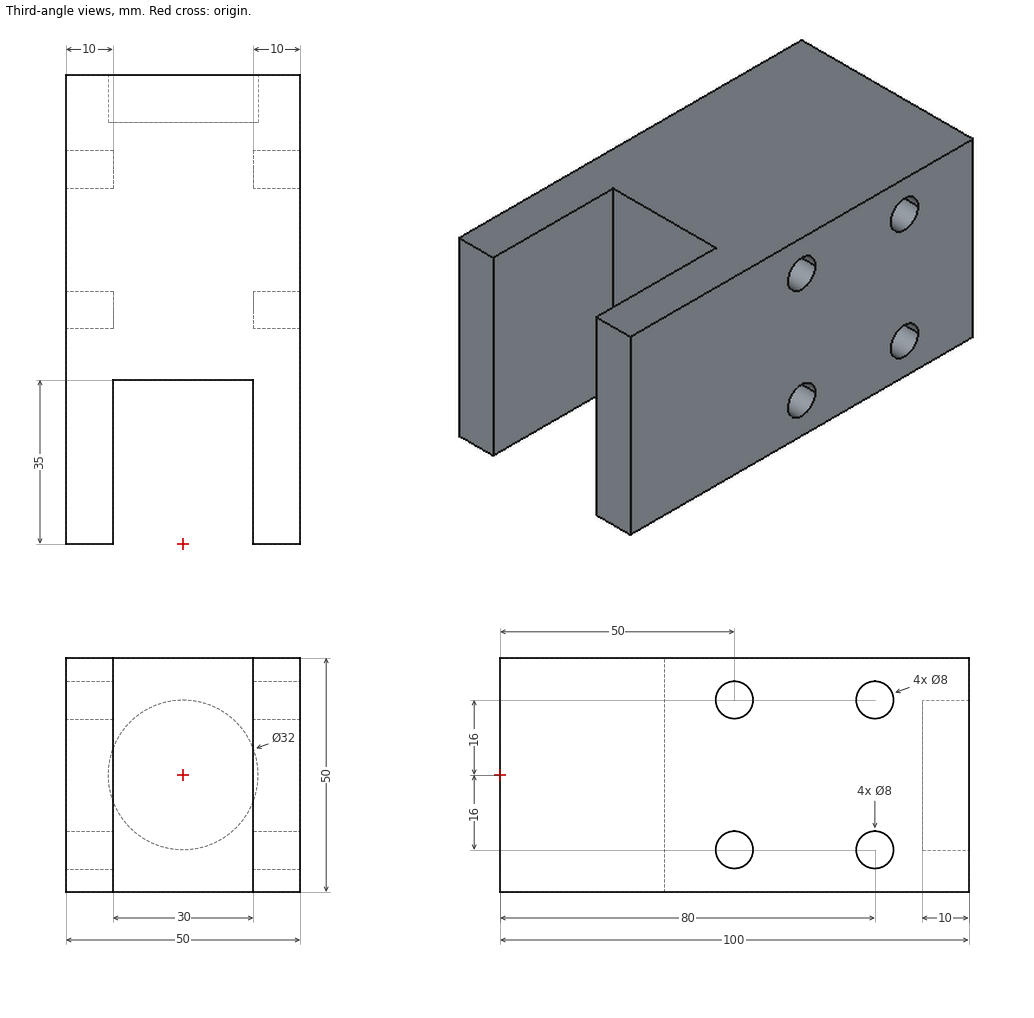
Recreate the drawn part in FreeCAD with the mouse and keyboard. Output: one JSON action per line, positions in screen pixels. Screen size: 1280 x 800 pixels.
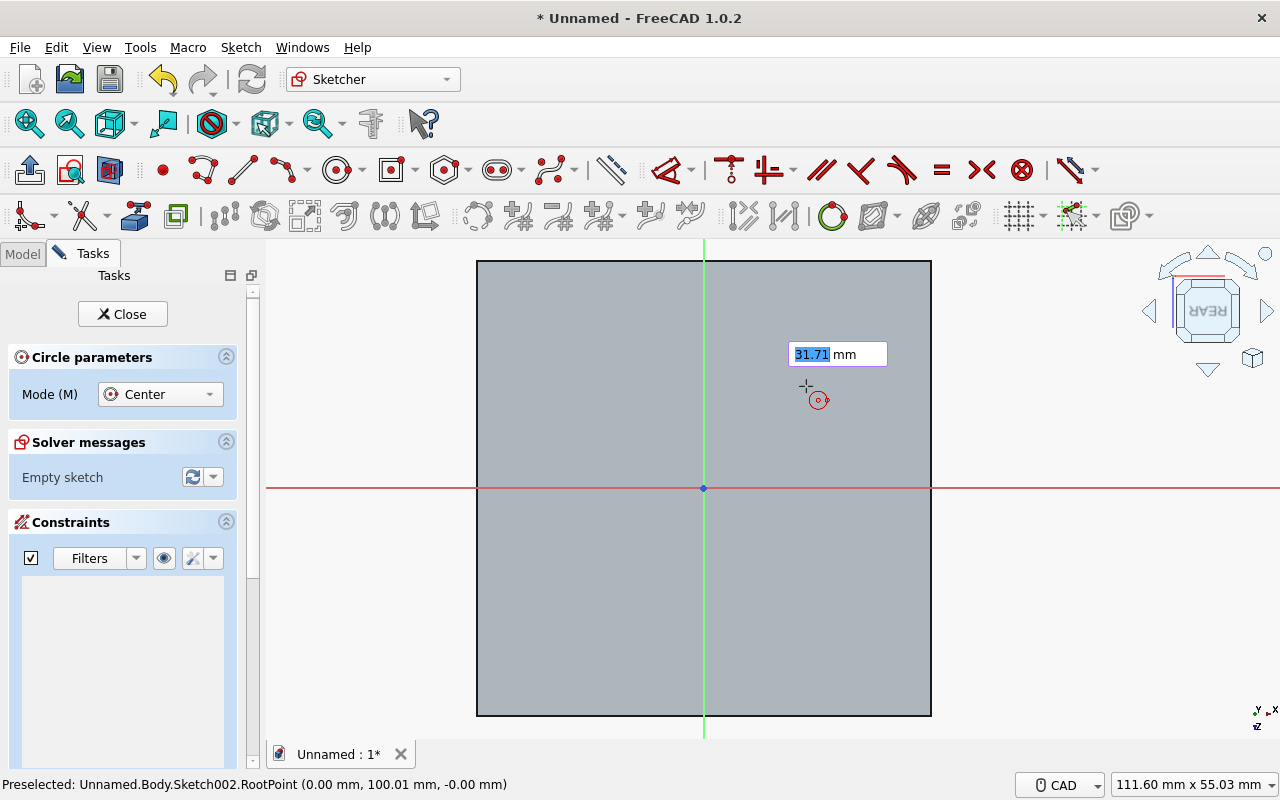
{"action": "type", "text": "32"}
{"action": "key", "text": "Return"}
{"action": "key", "text": "Escape"}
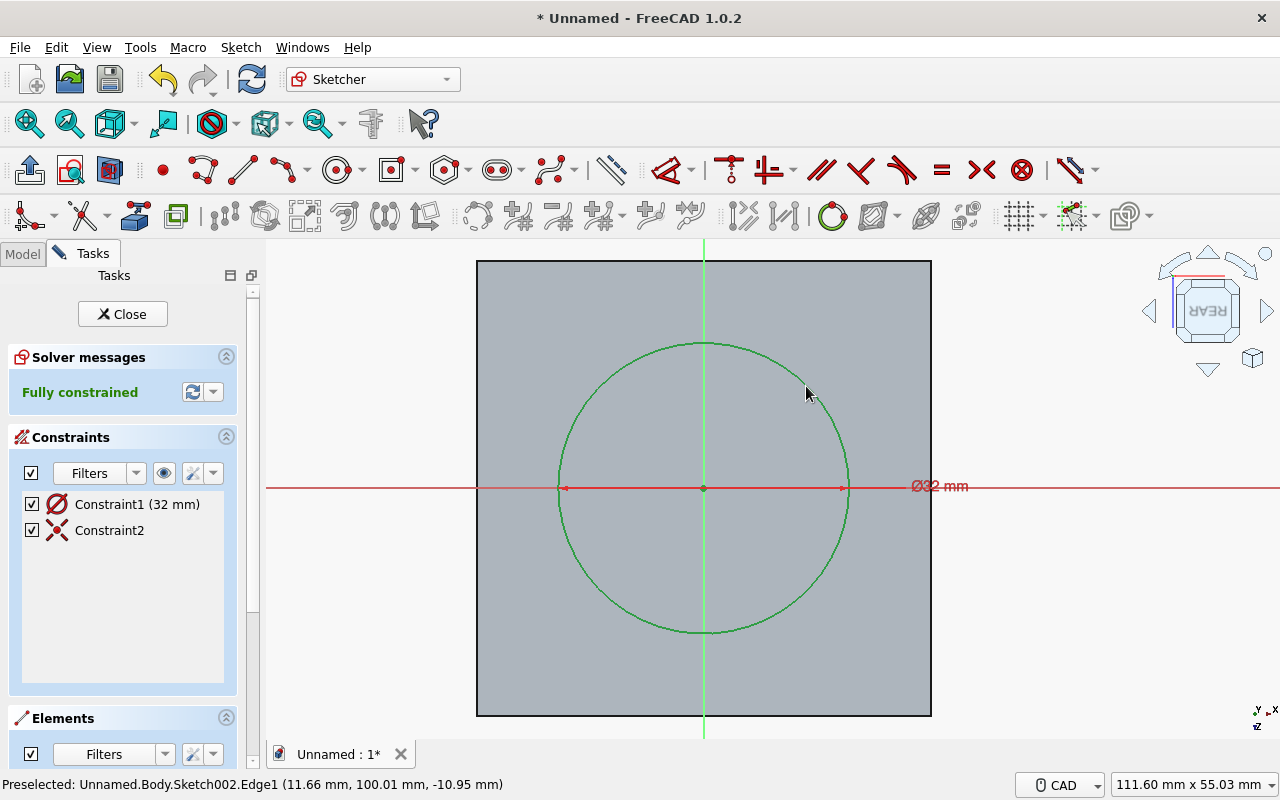
{"action": "left_click", "coordinate": [123, 314]}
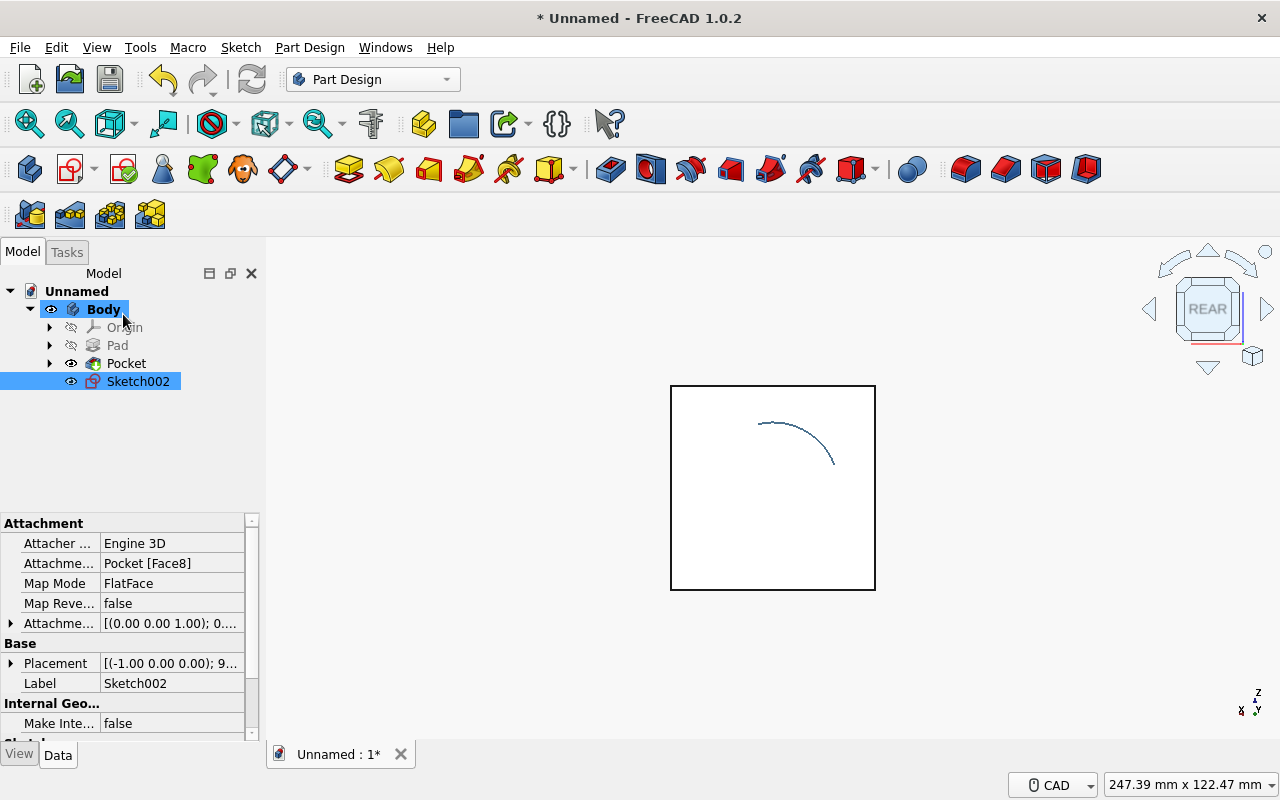
{"action": "left_click", "coordinate": [612, 170]}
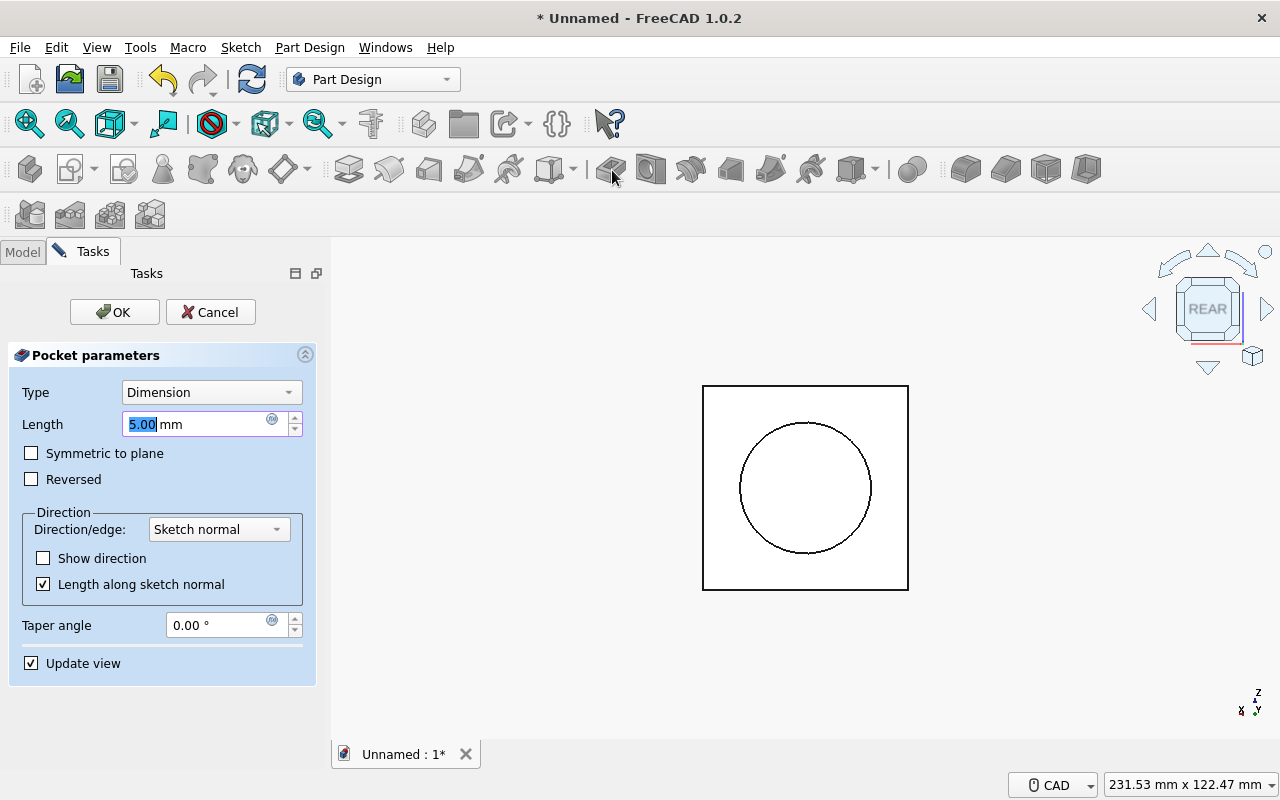
{"action": "type", "text": "10"}
{"action": "key", "text": "Tab"}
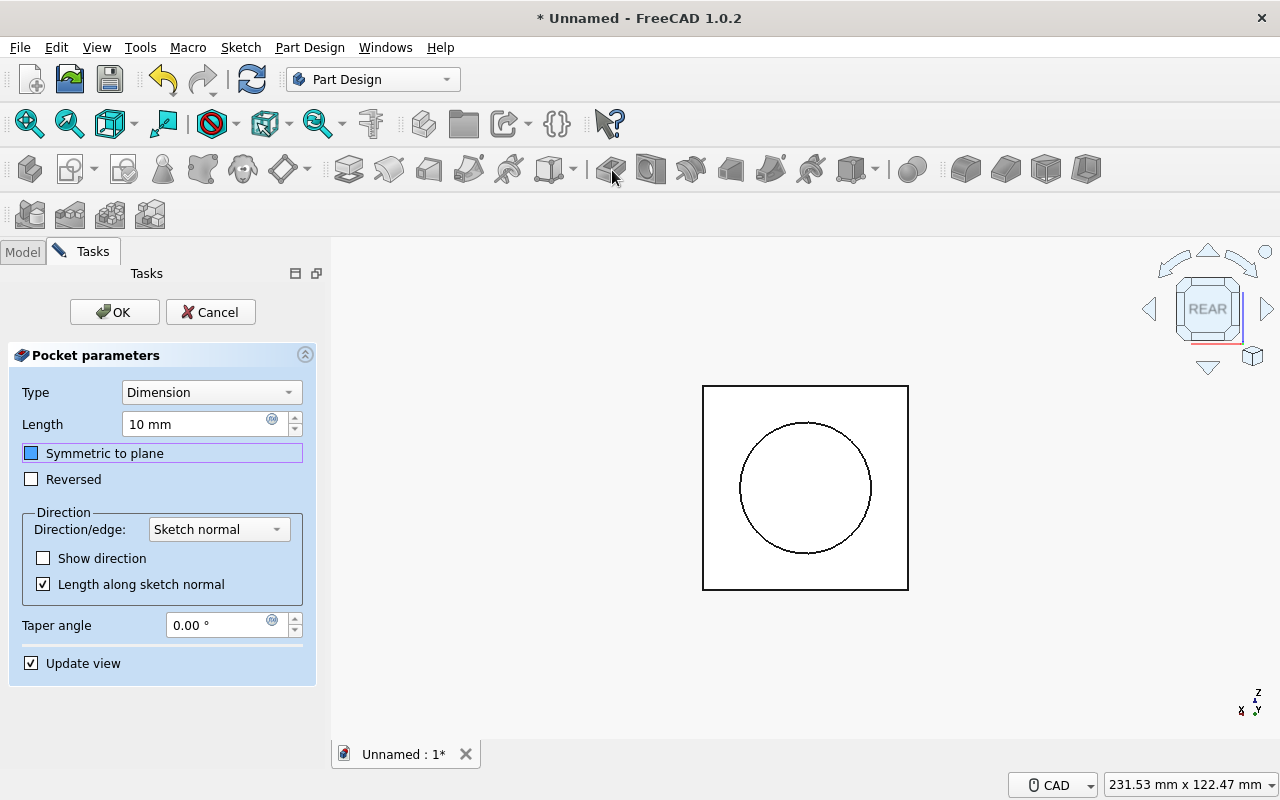
{"action": "left_click", "coordinate": [115, 312]}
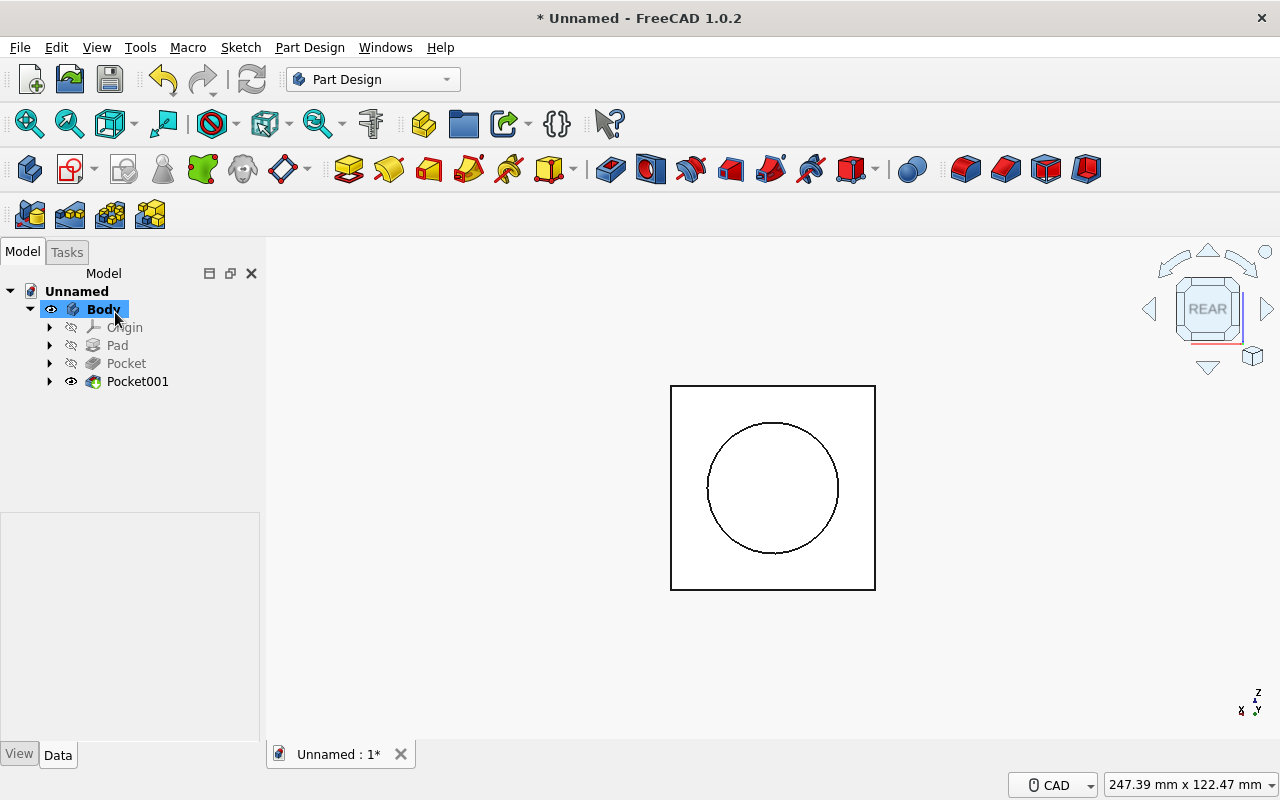
{"action": "left_click", "coordinate": [30, 124]}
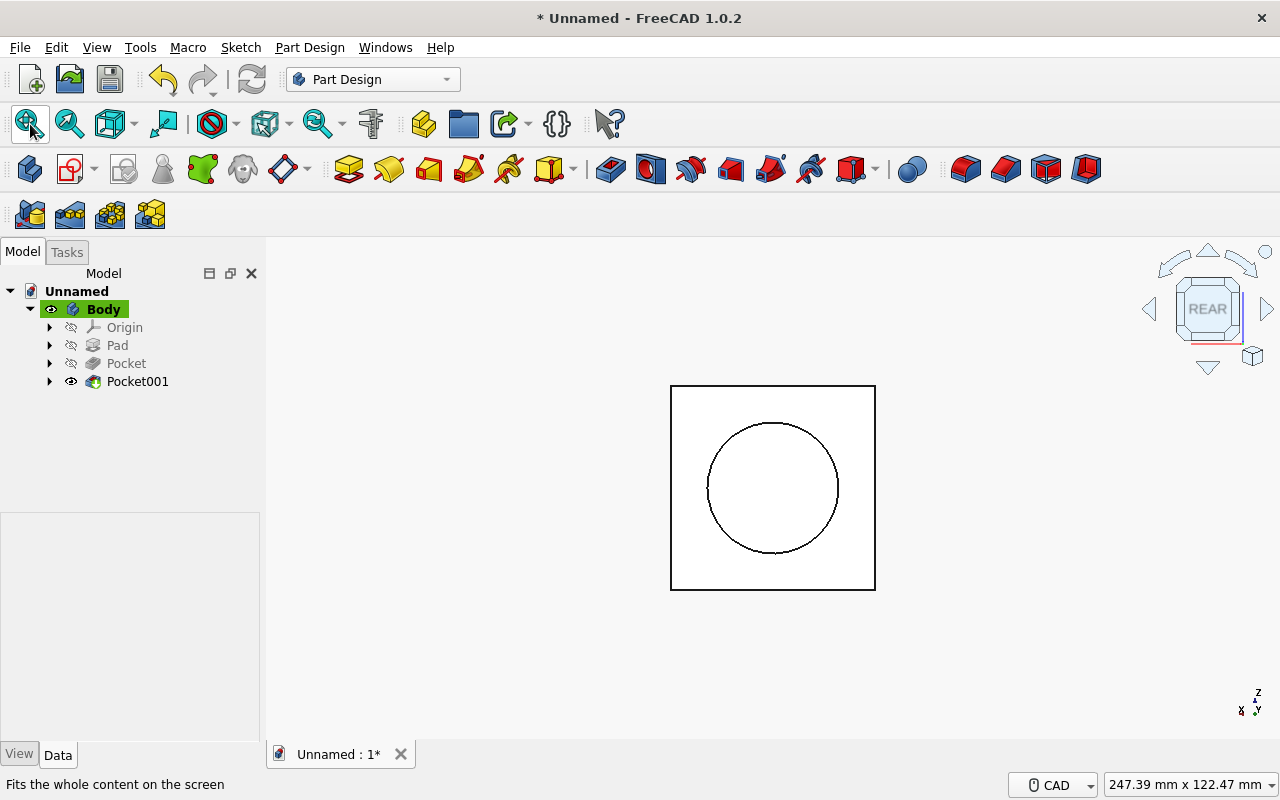
{"action": "key", "text": "6"}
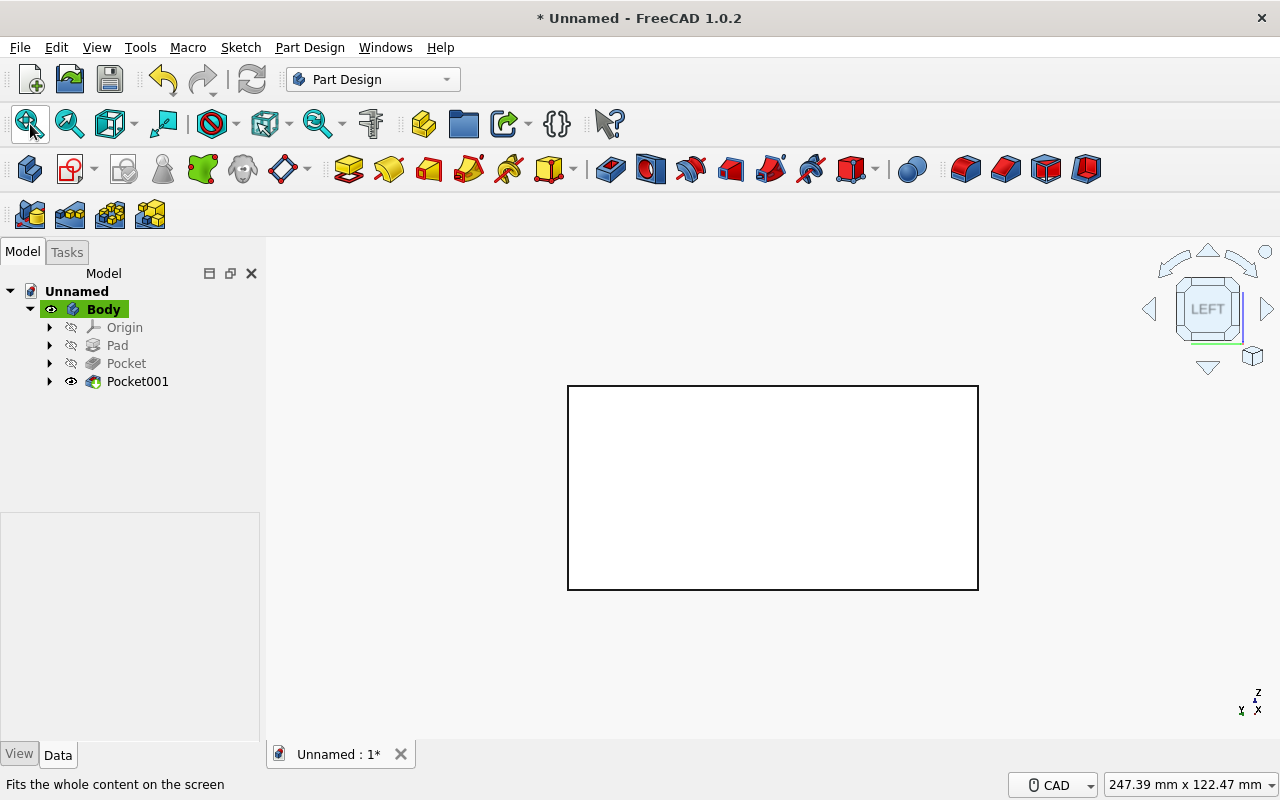
{"action": "left_click", "coordinate": [30, 124]}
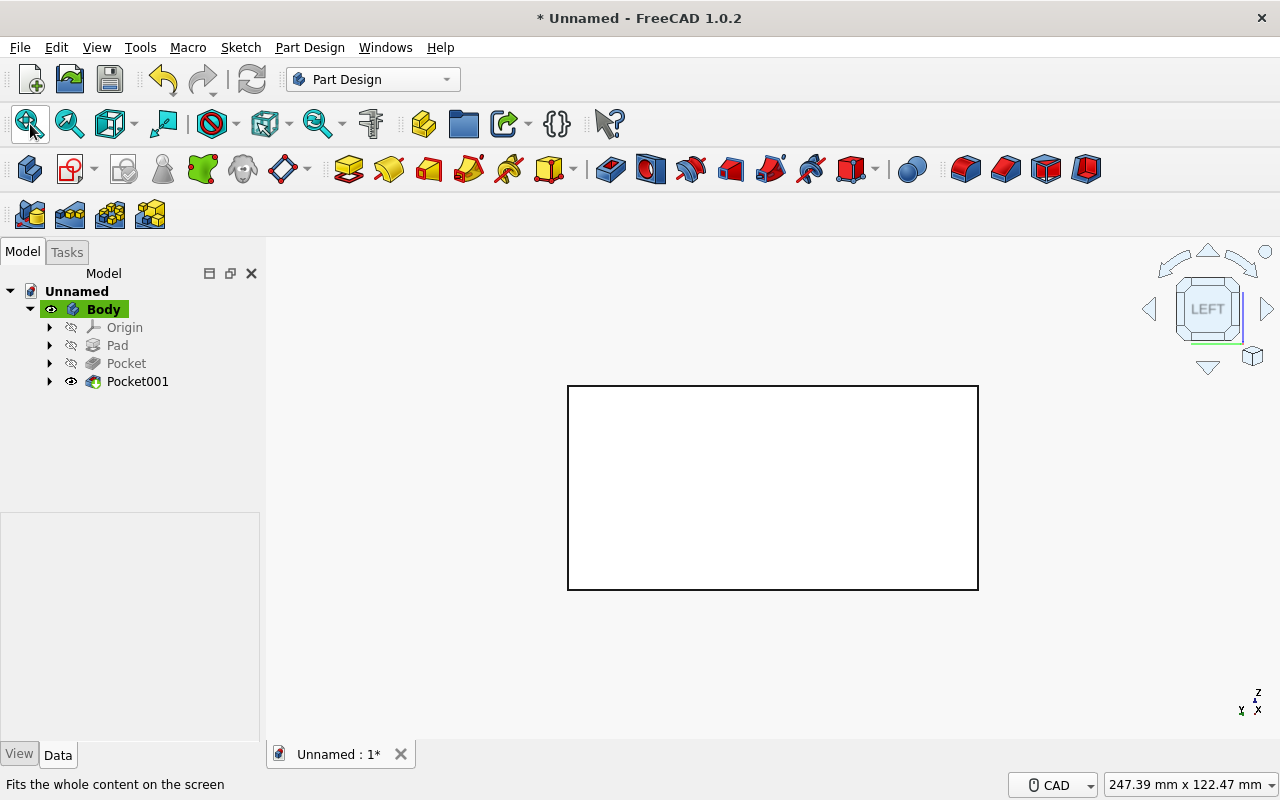
{"action": "left_click", "coordinate": [714, 487]}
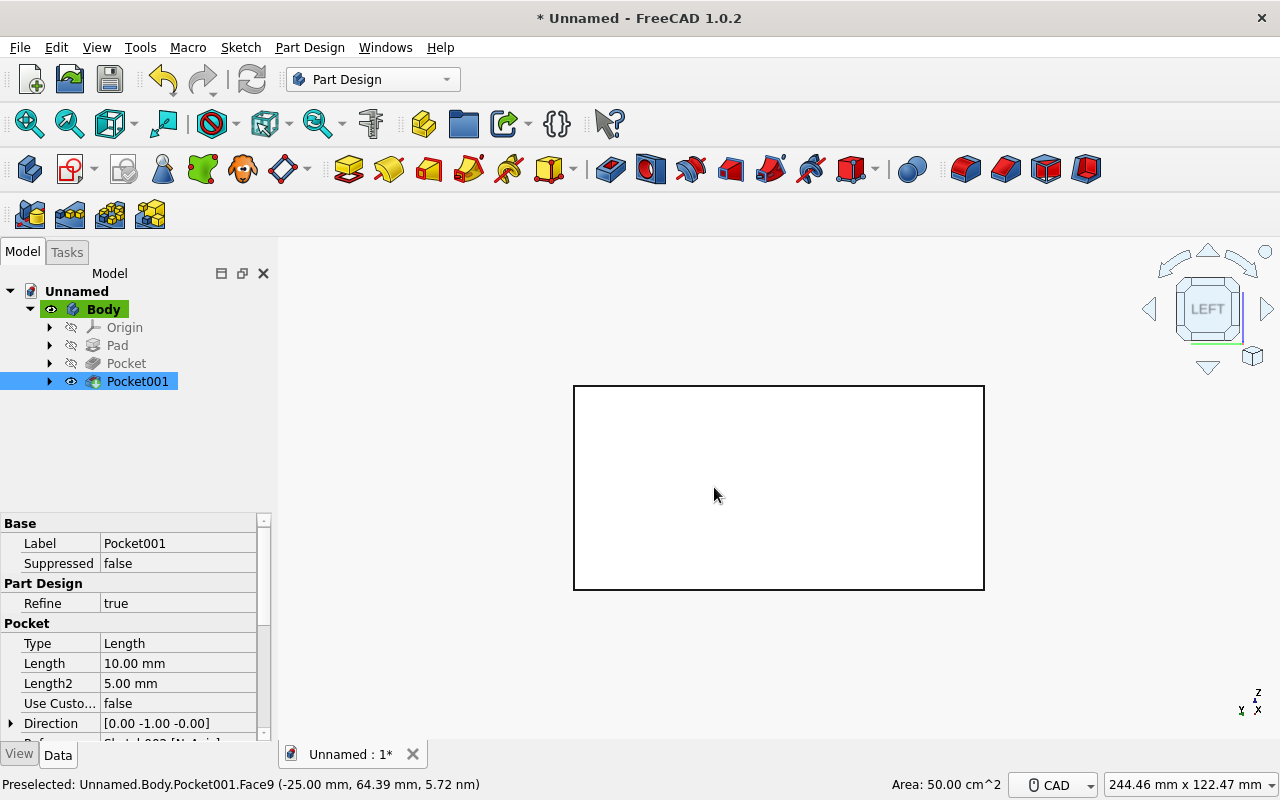
{"action": "left_click", "coordinate": [70, 170]}